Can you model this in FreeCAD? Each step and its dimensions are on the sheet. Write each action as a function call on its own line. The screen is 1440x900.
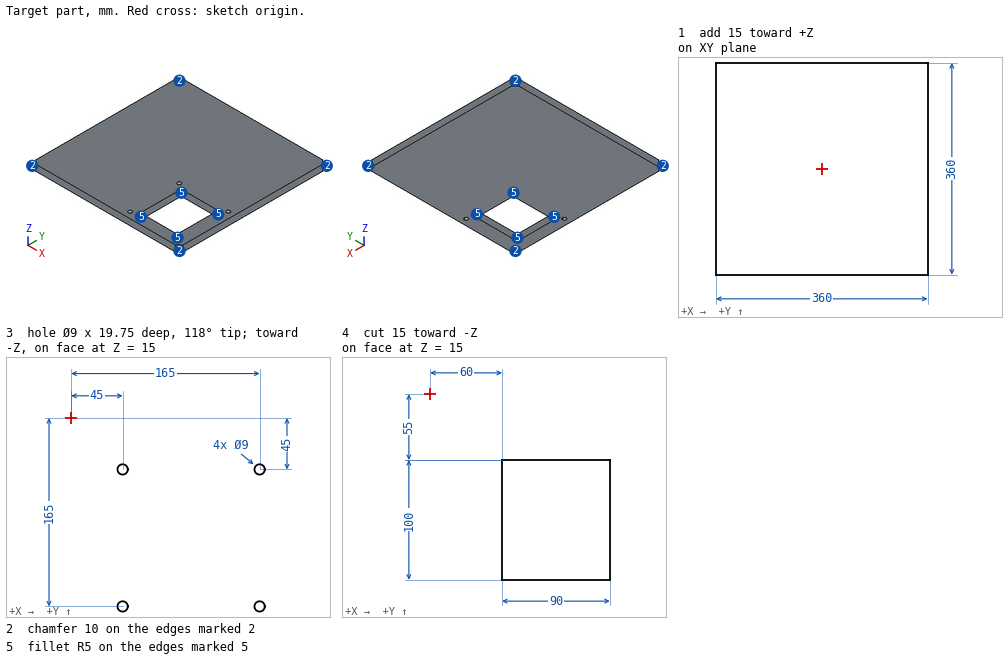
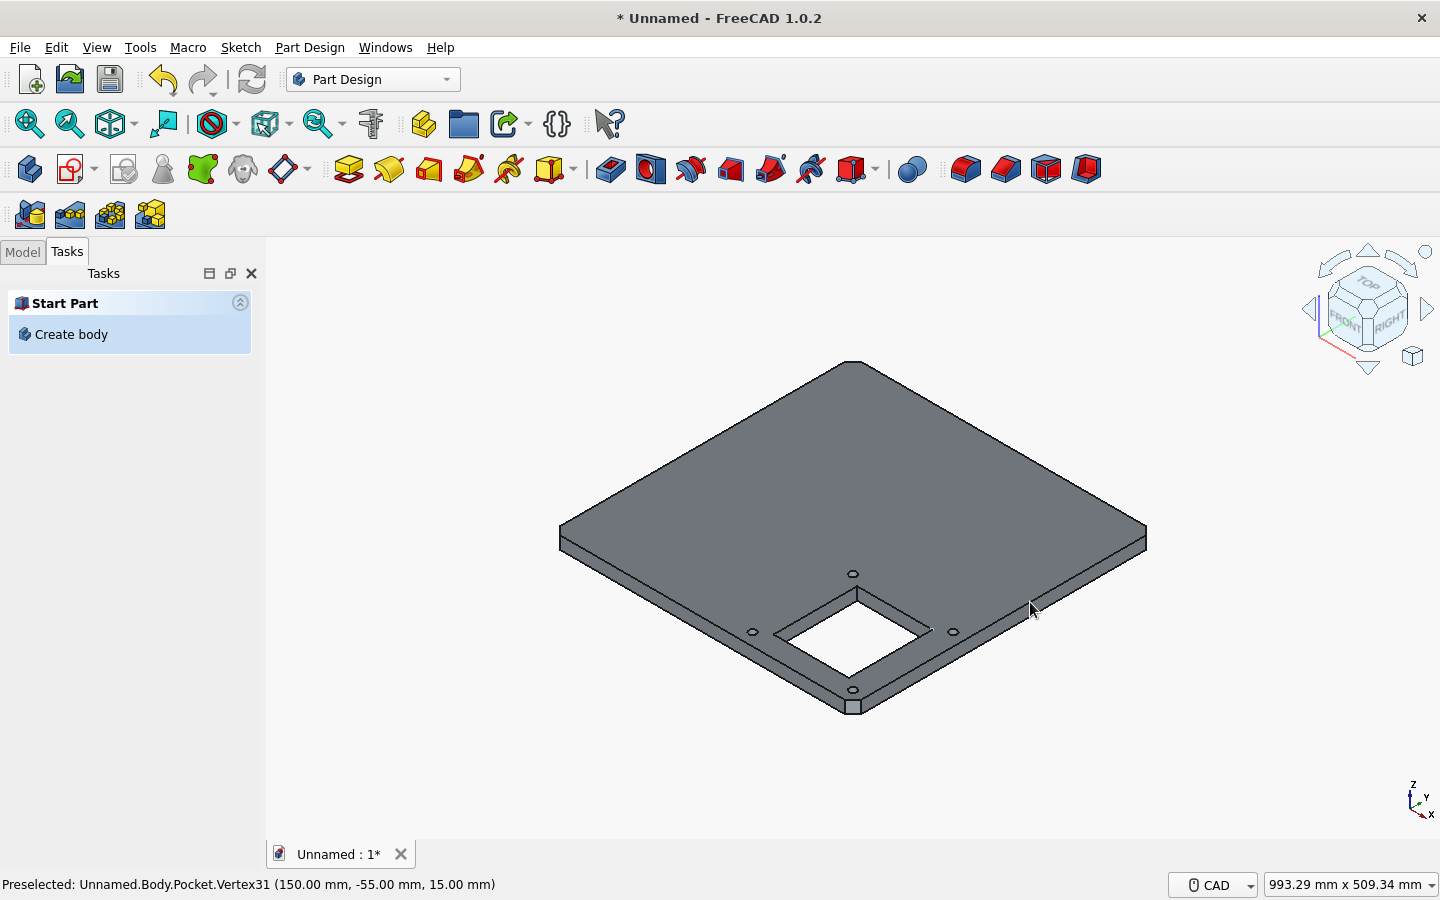
scroll(932, 636, up, 5)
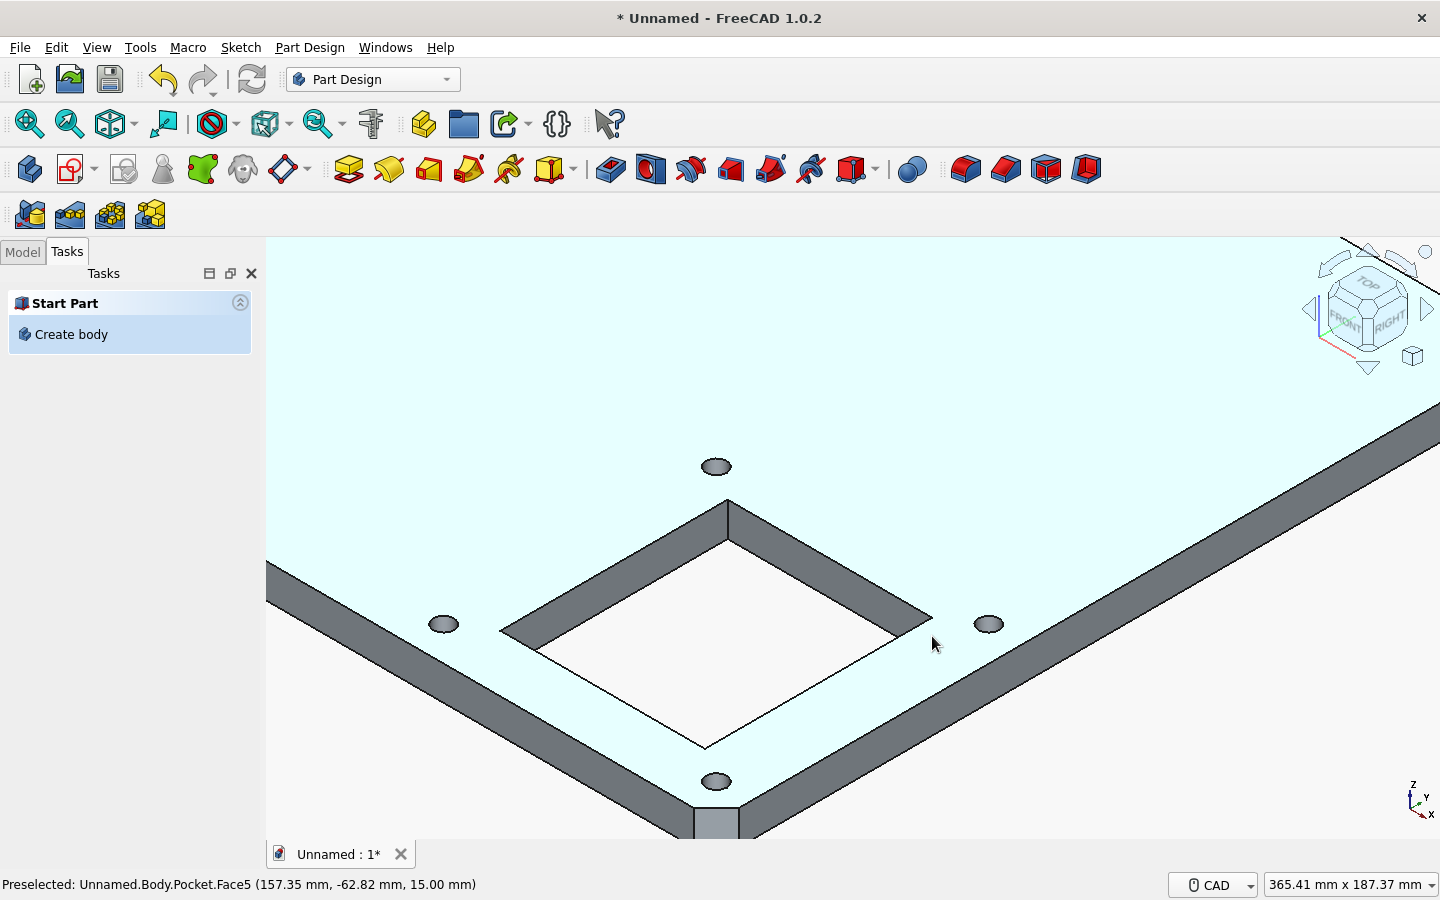
click(30, 124)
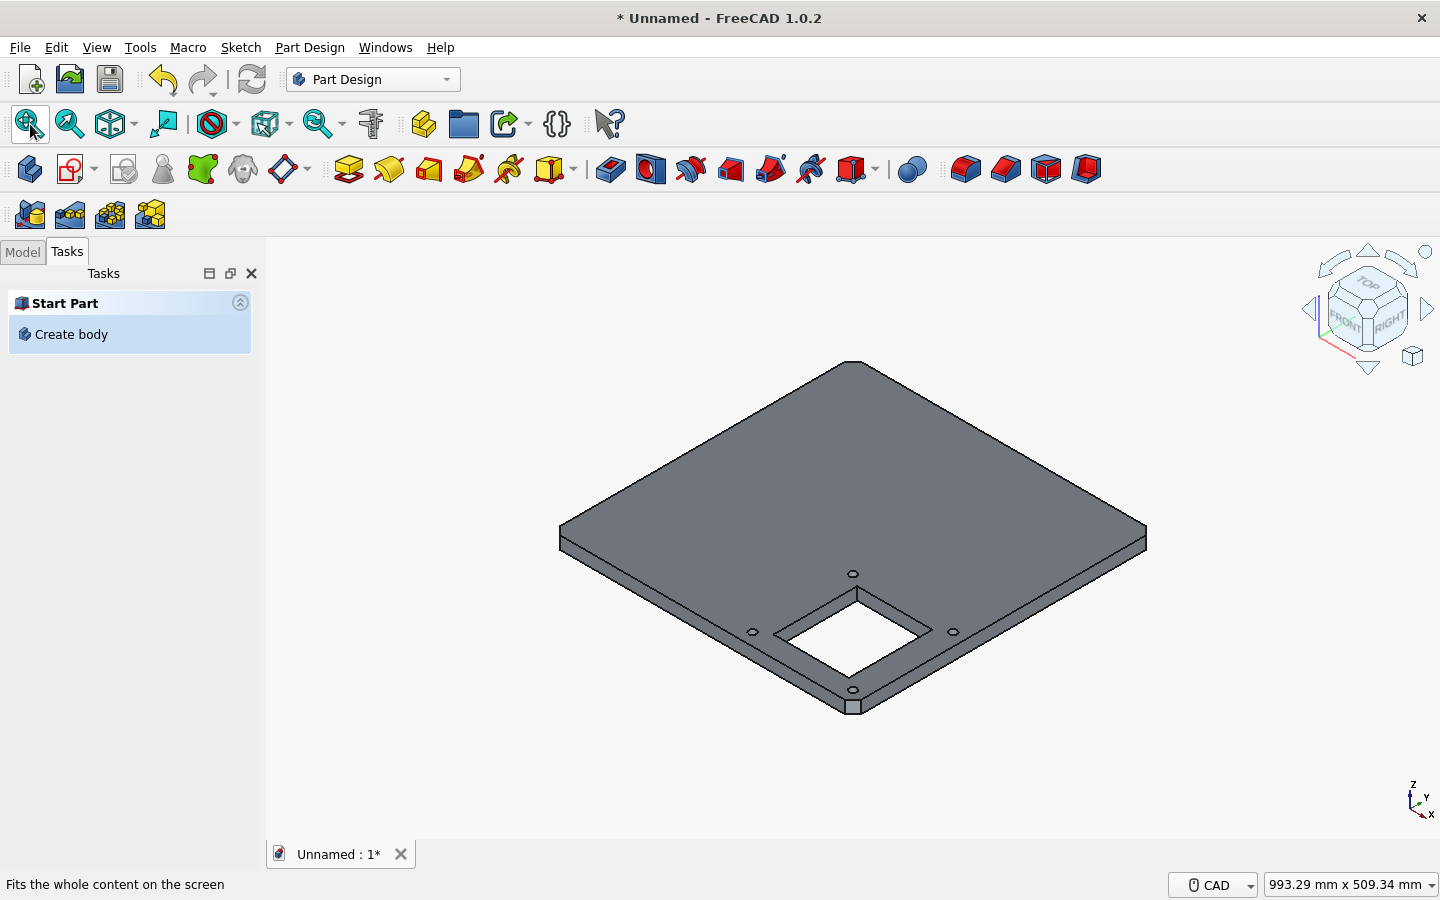
key(1)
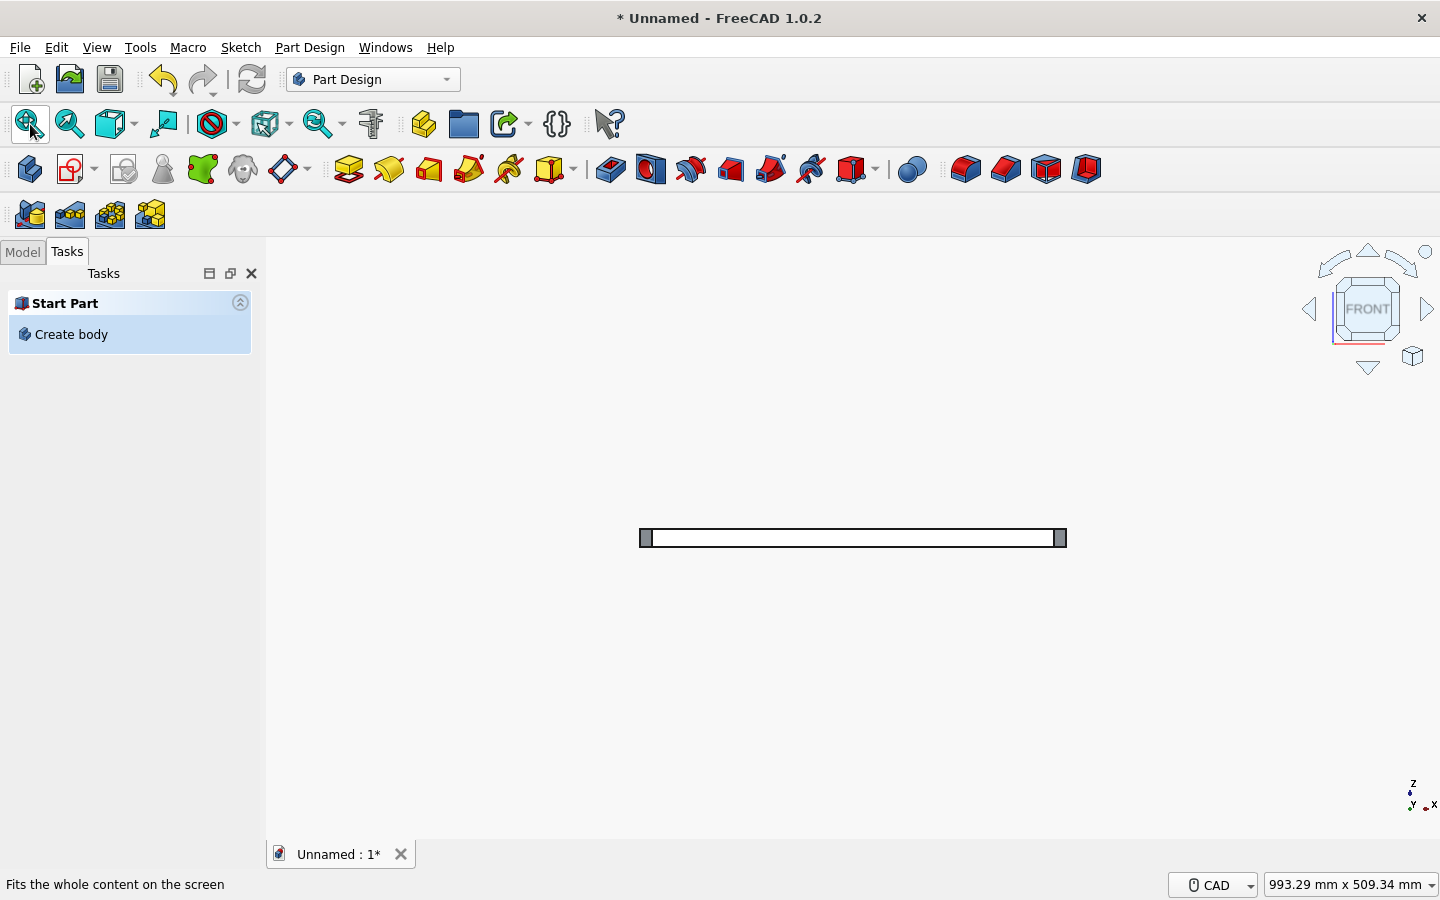
click(30, 124)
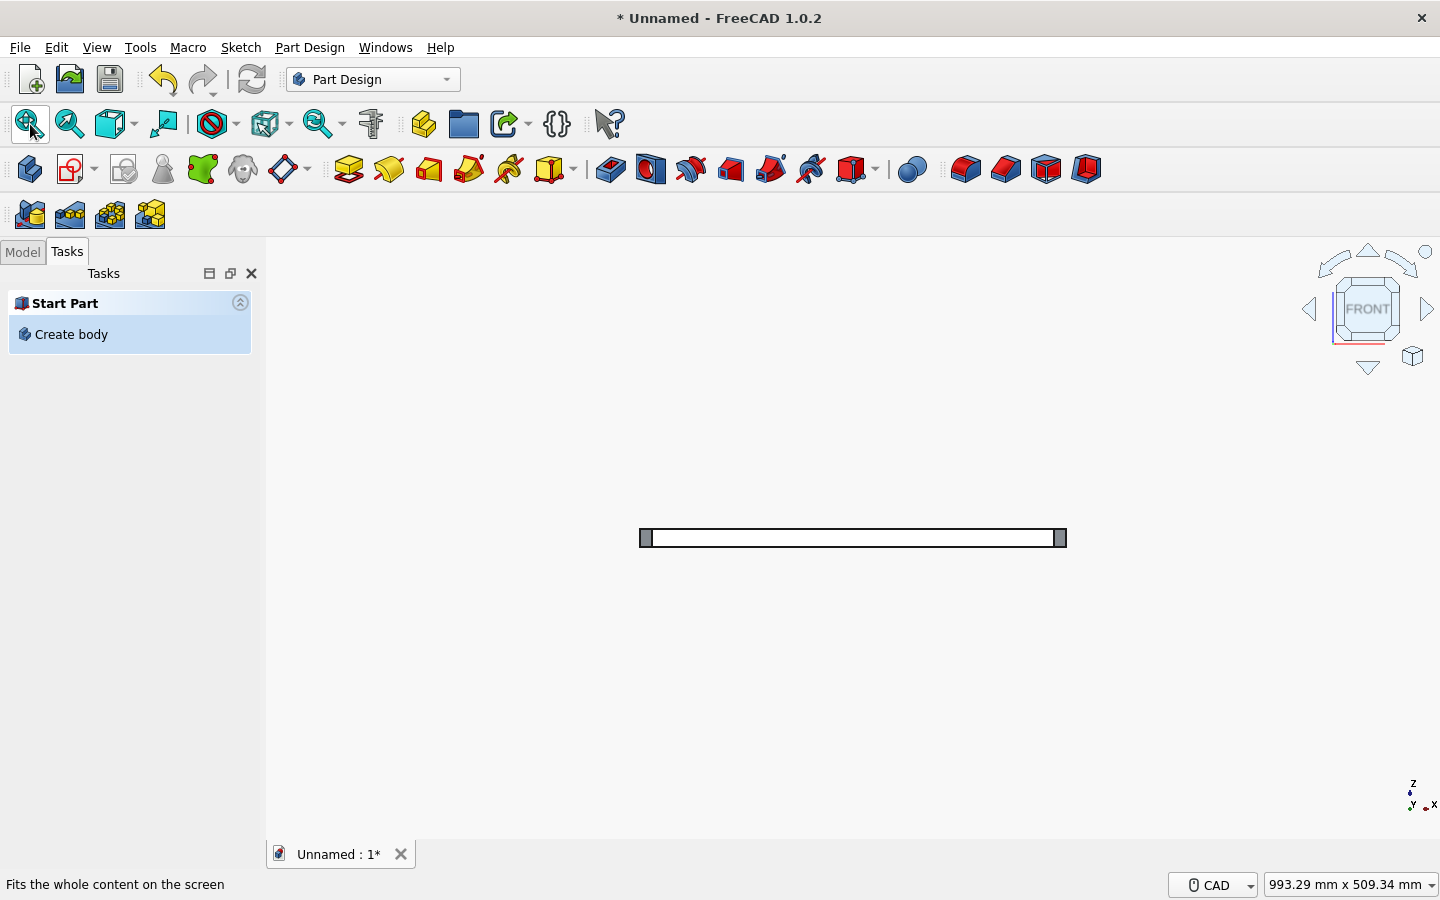
scroll(1030, 537, up, 5)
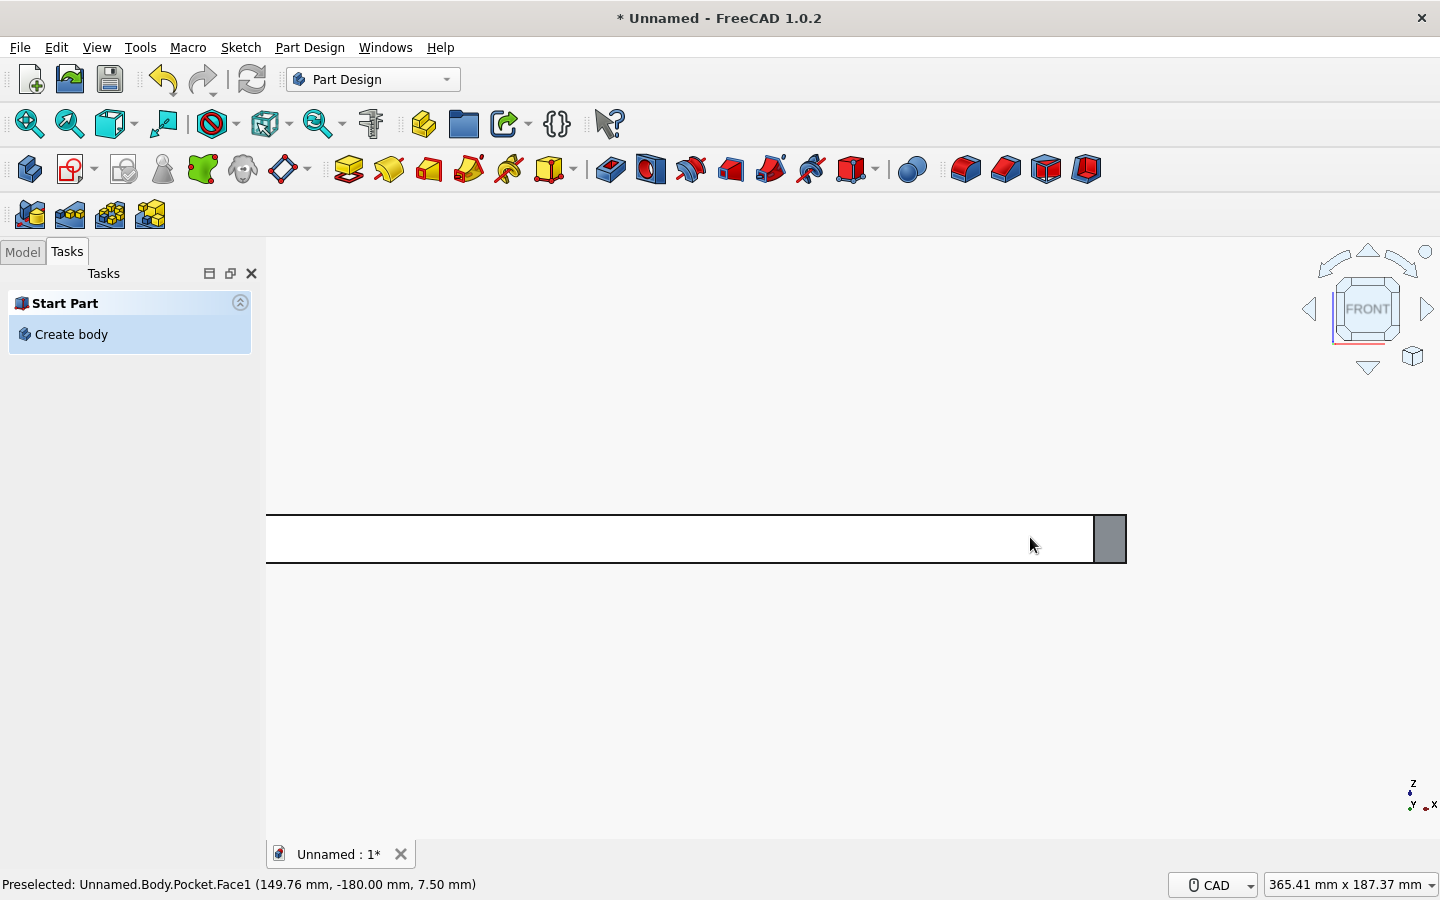
click(30, 124)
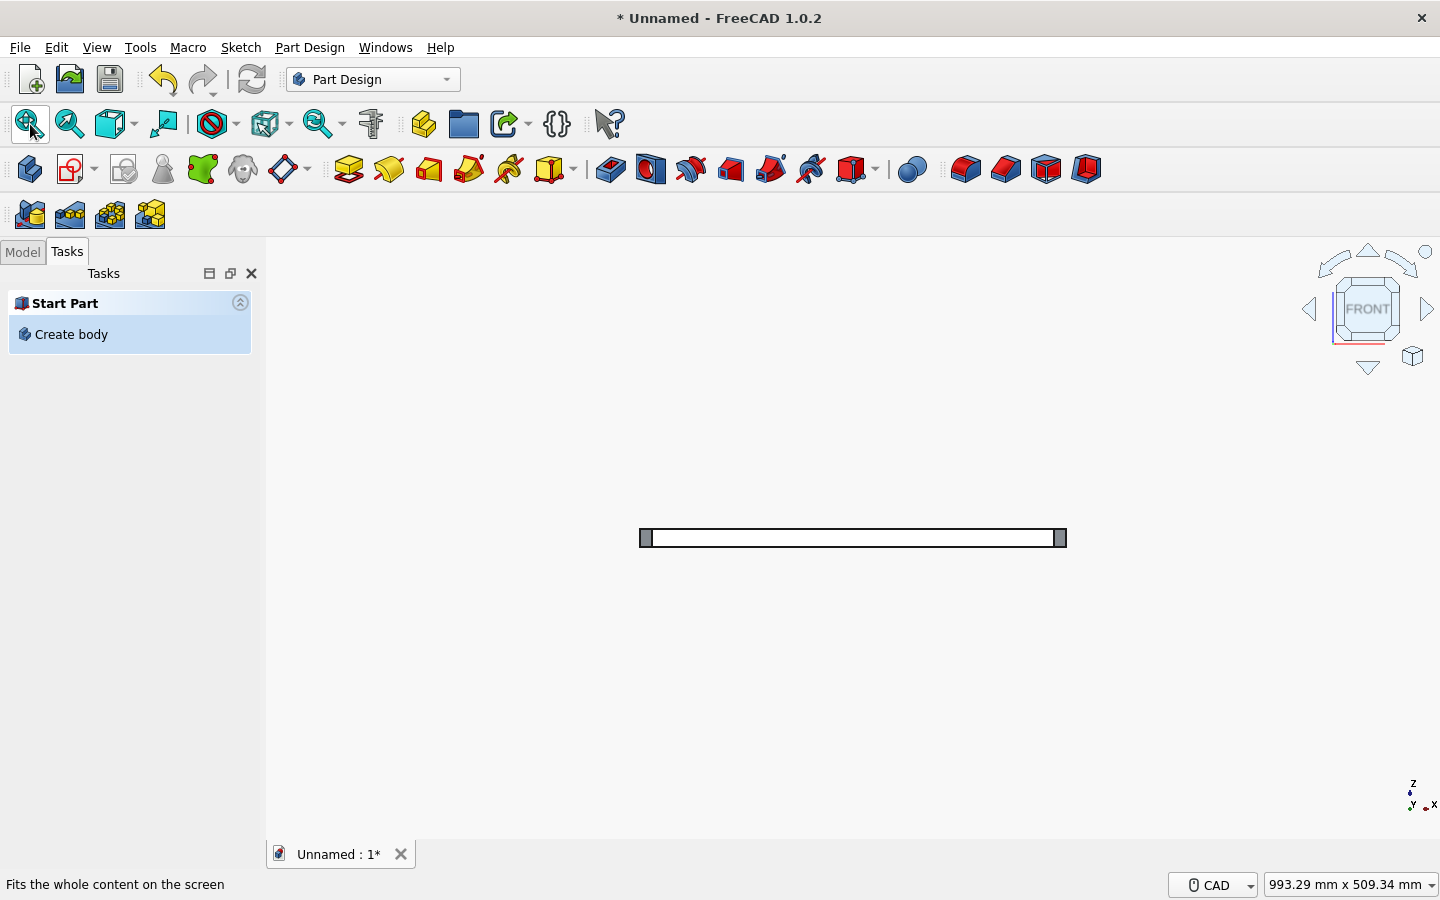
key(3)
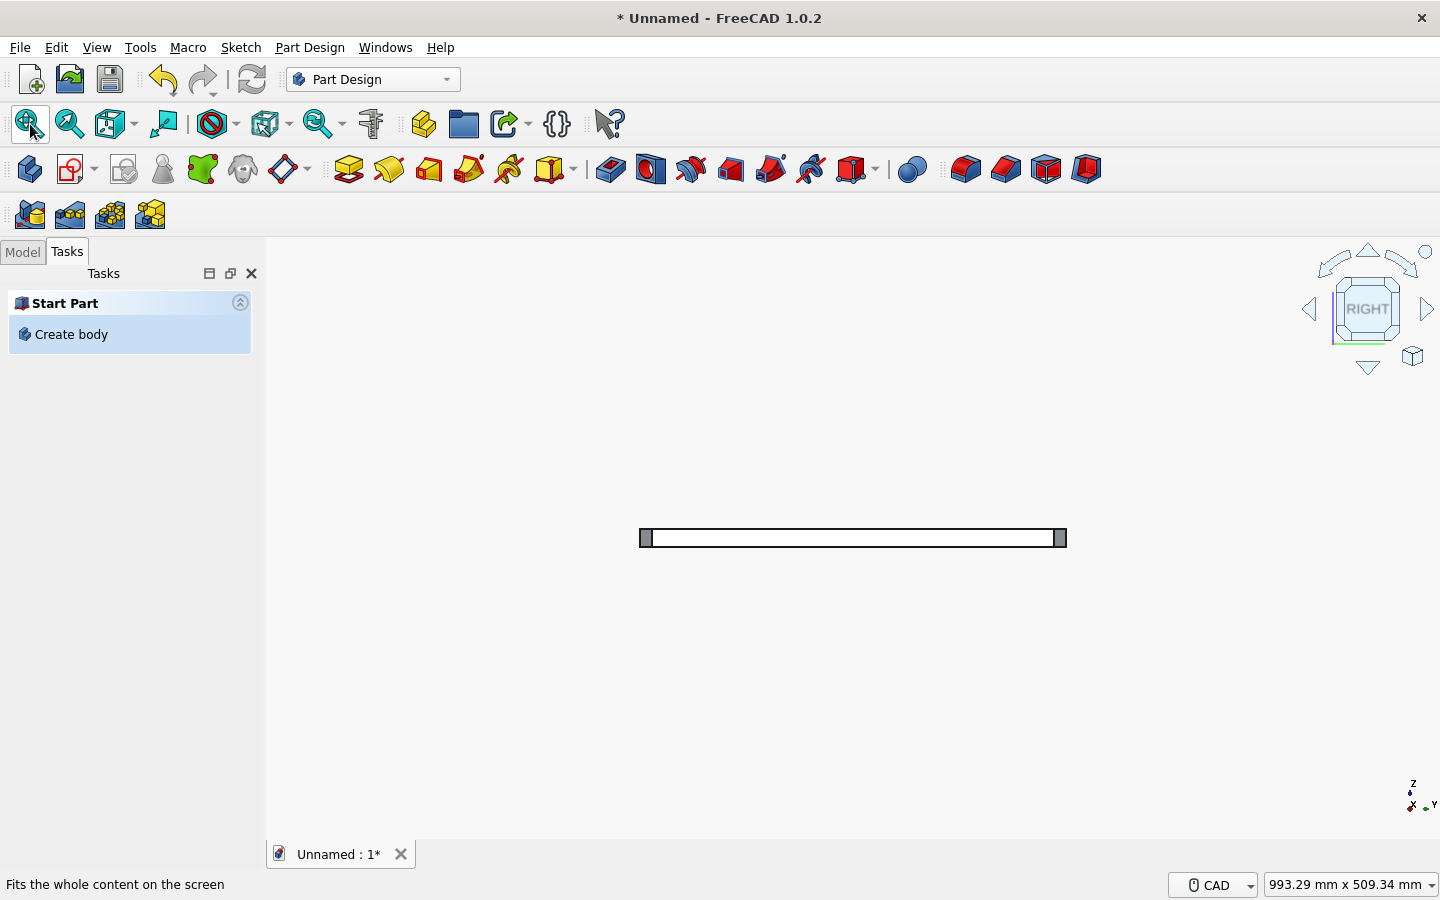
key(v)
key(f)